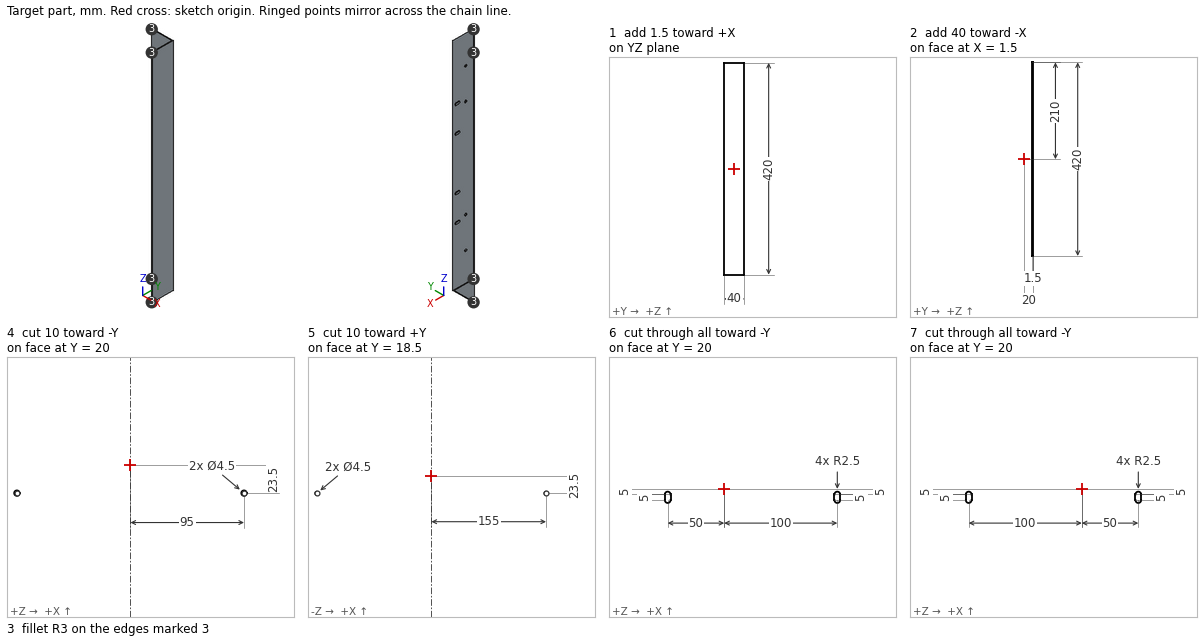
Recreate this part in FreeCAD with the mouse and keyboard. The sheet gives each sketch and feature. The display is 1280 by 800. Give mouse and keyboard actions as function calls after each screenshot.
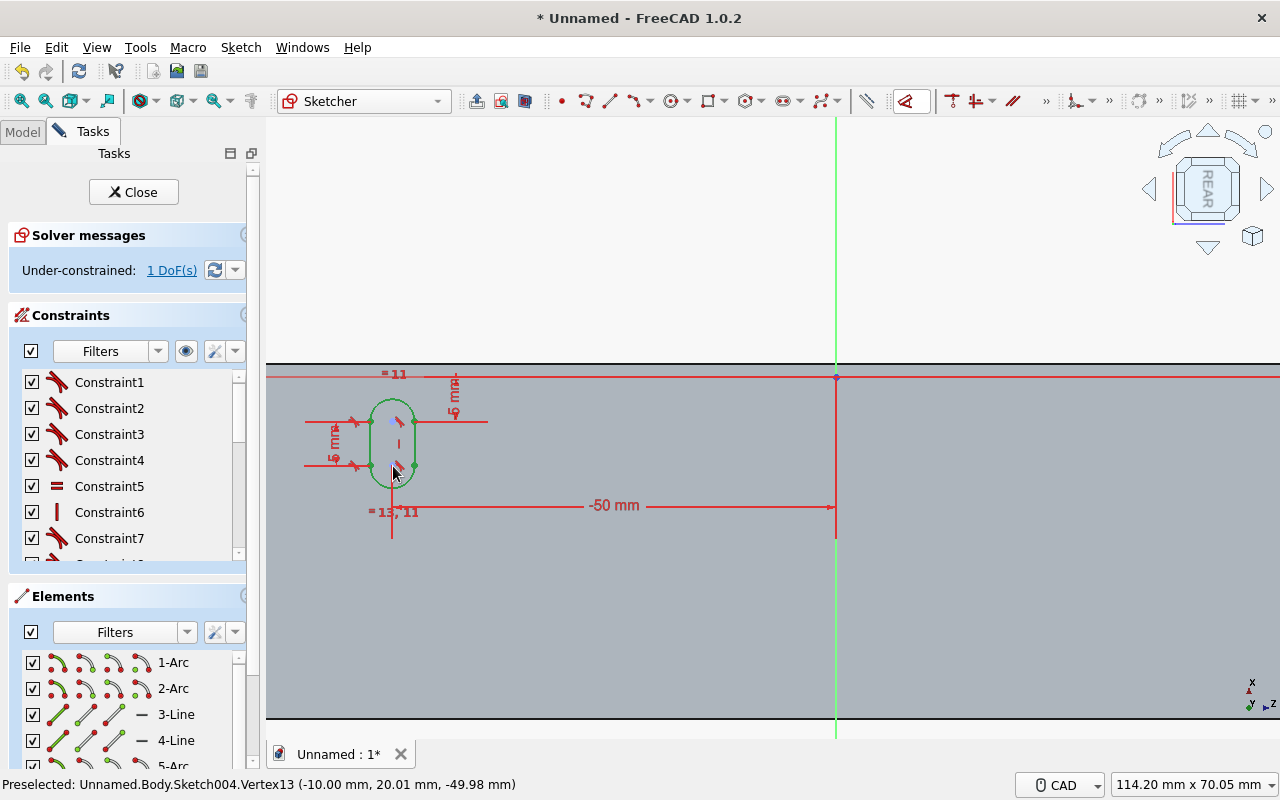
scroll(416, 424, down, 4)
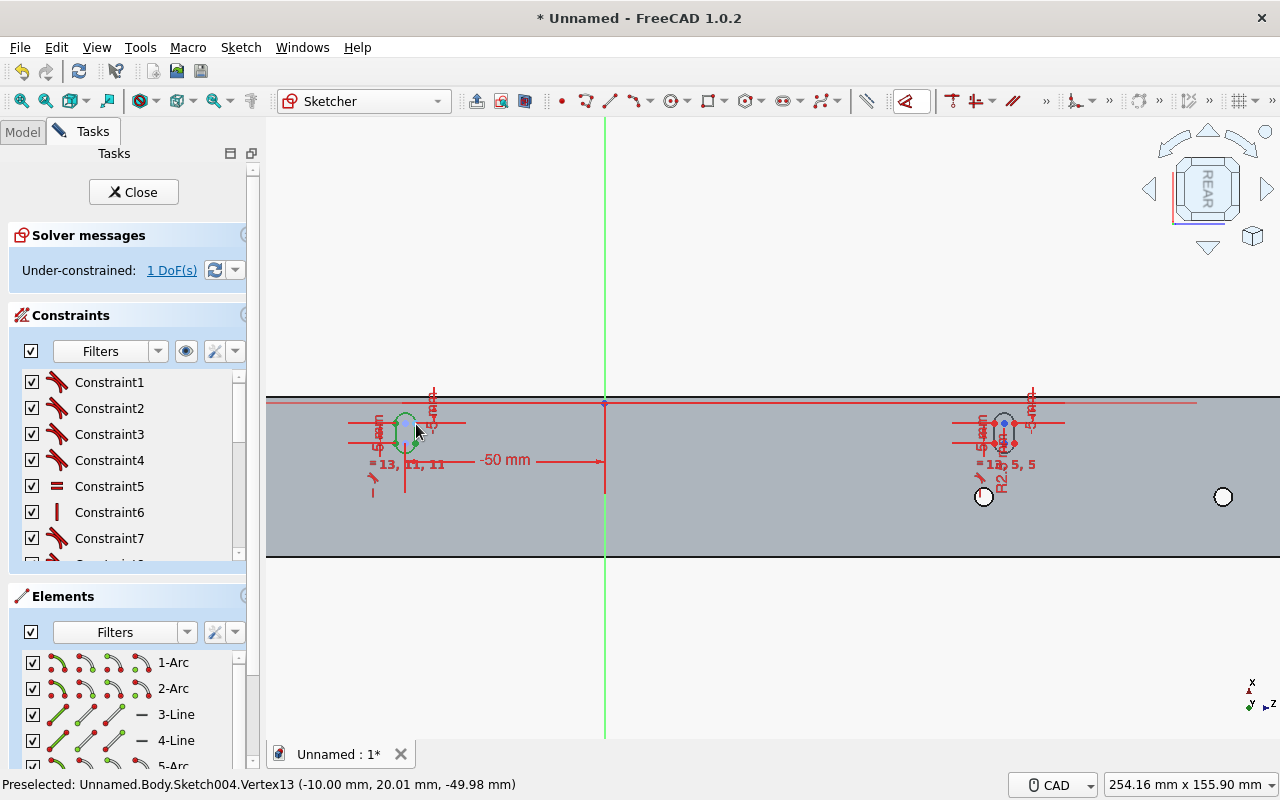
scroll(1004, 443, up, 2)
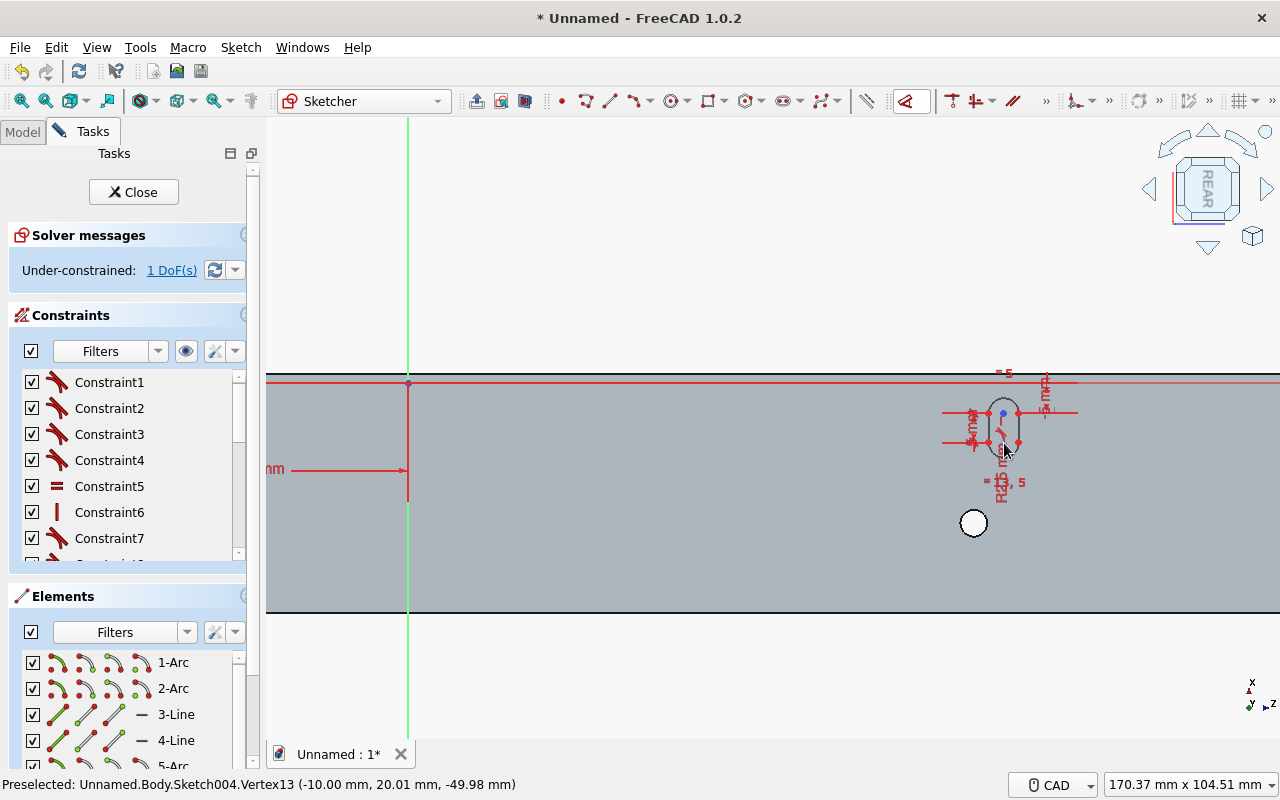
click(1004, 443)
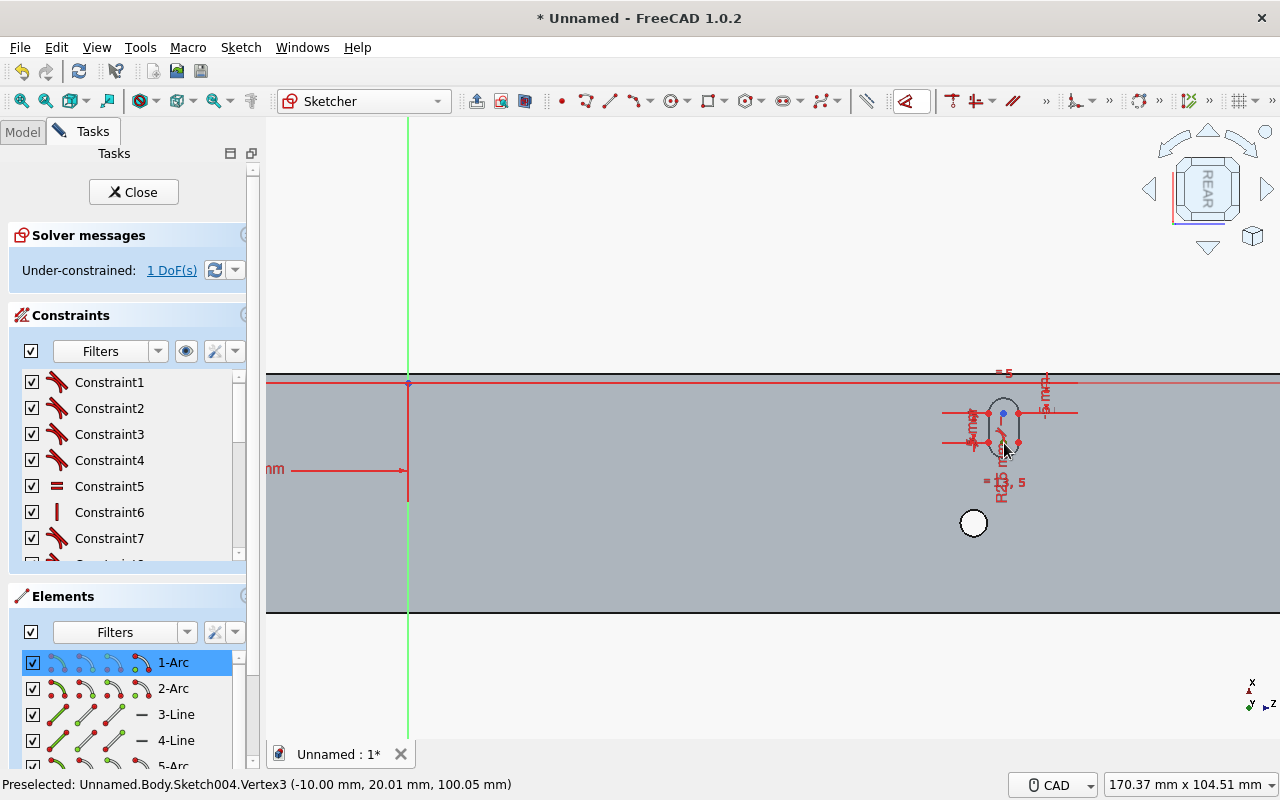
key(l)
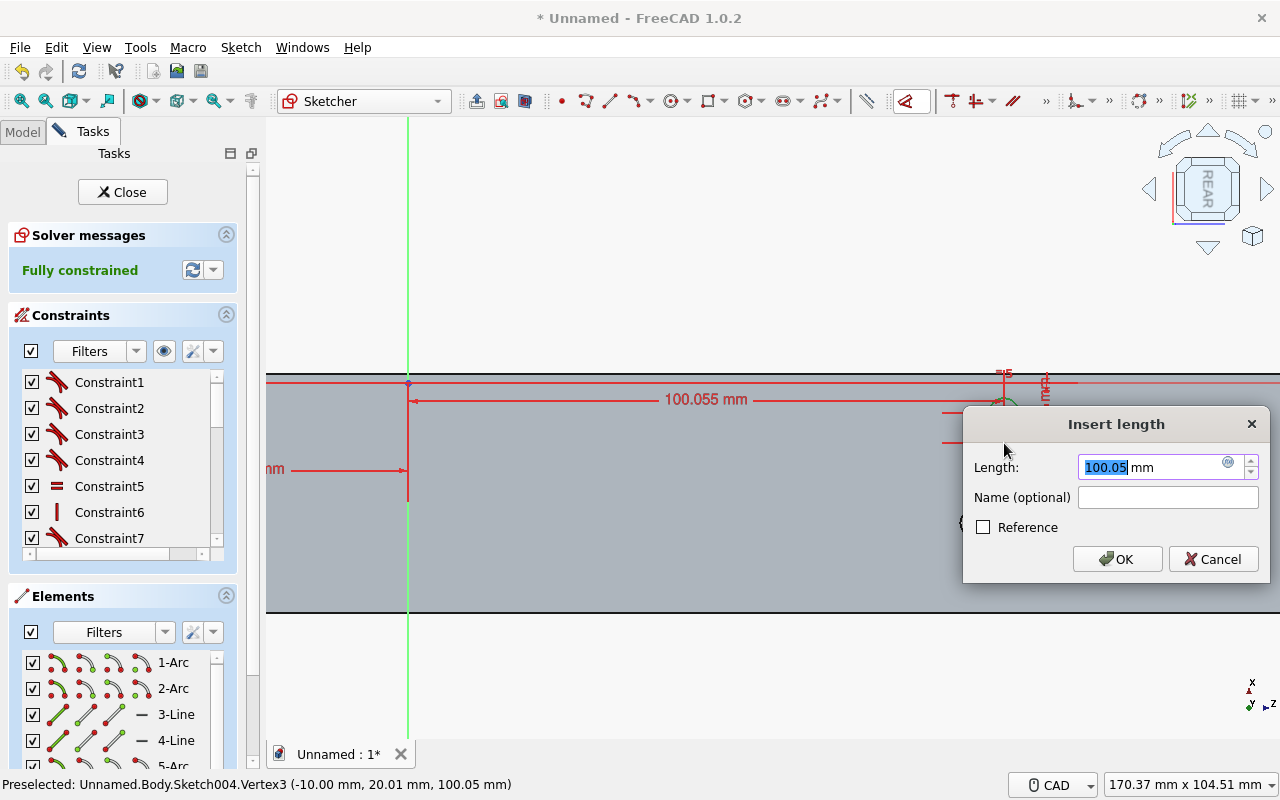
text(100)
key(Return)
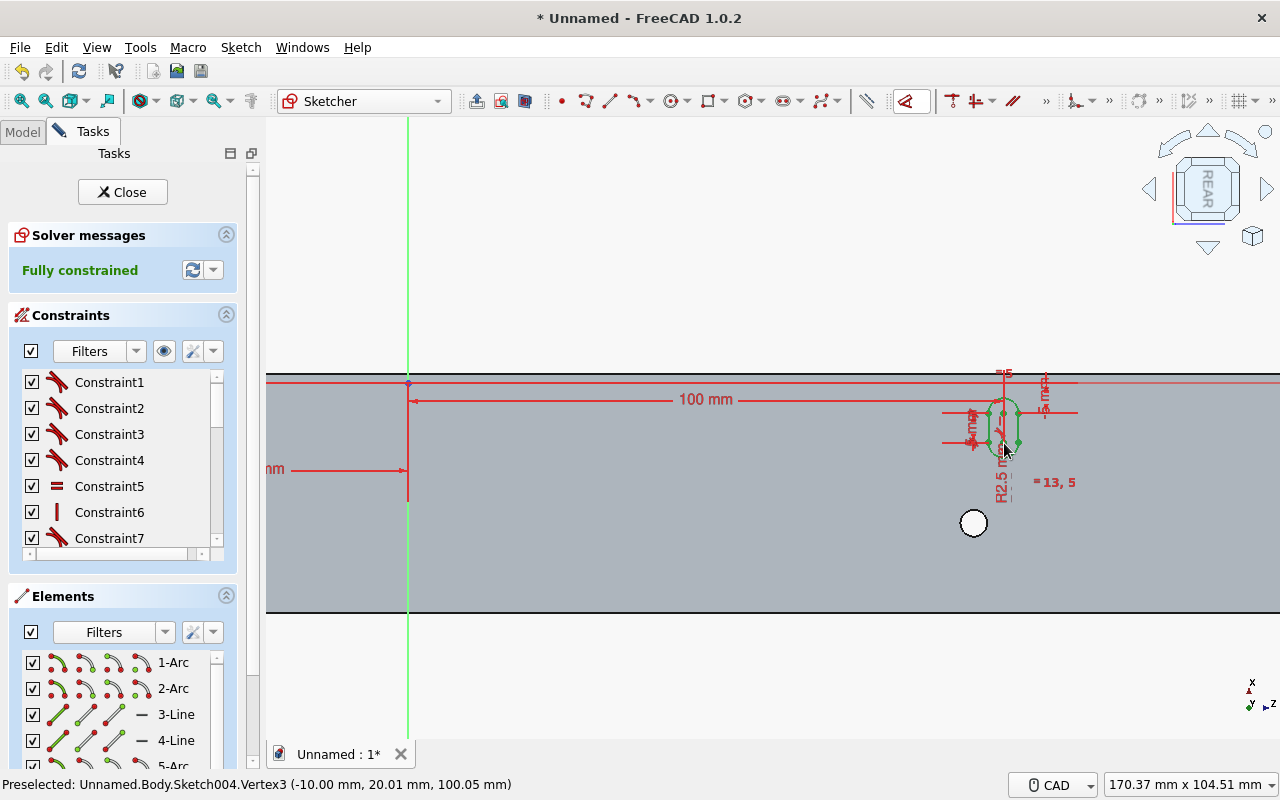
click(123, 192)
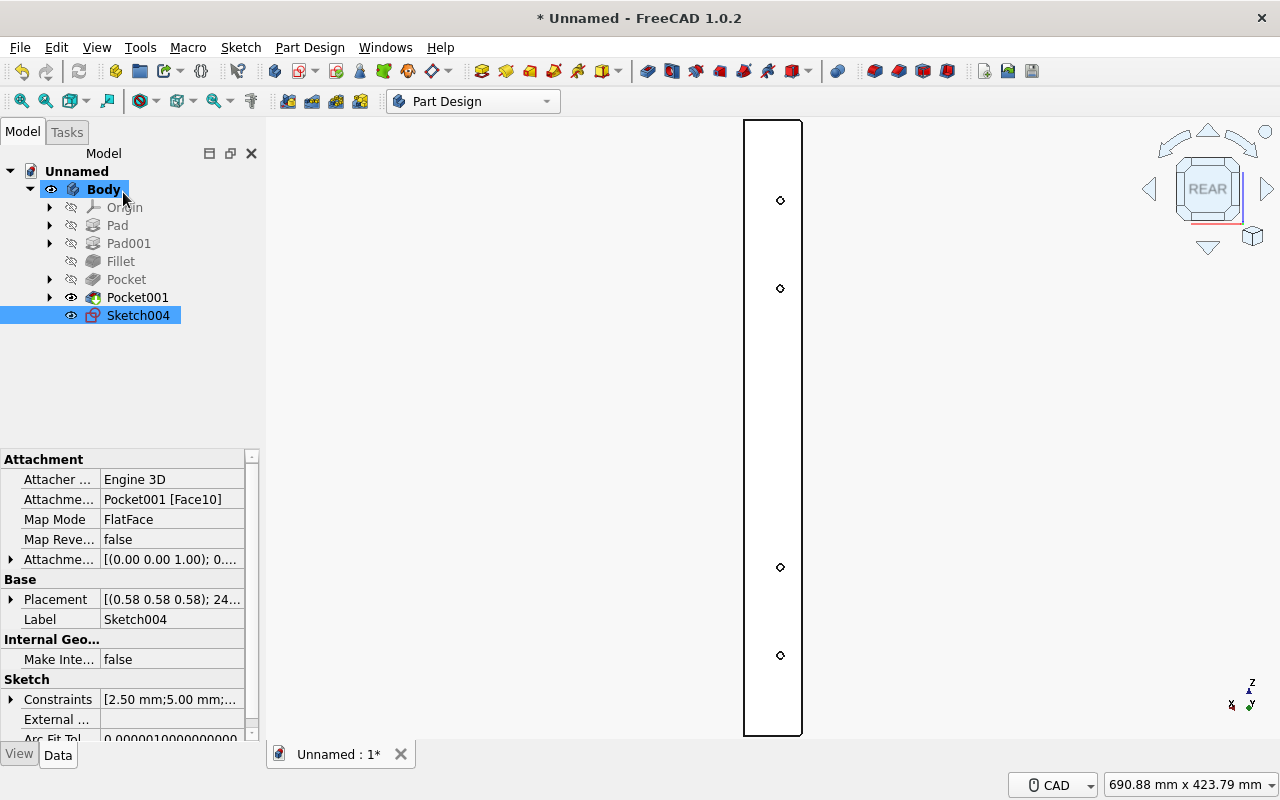
click(648, 72)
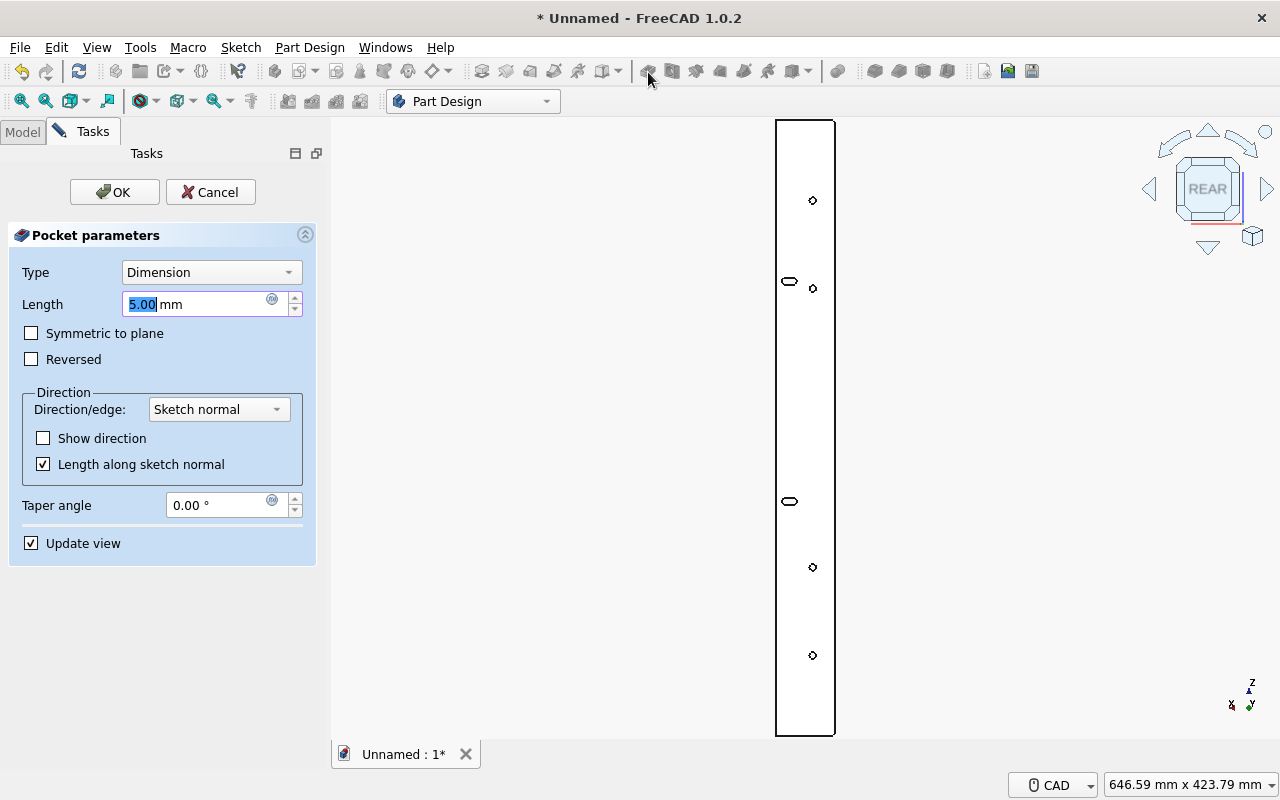
click(212, 272)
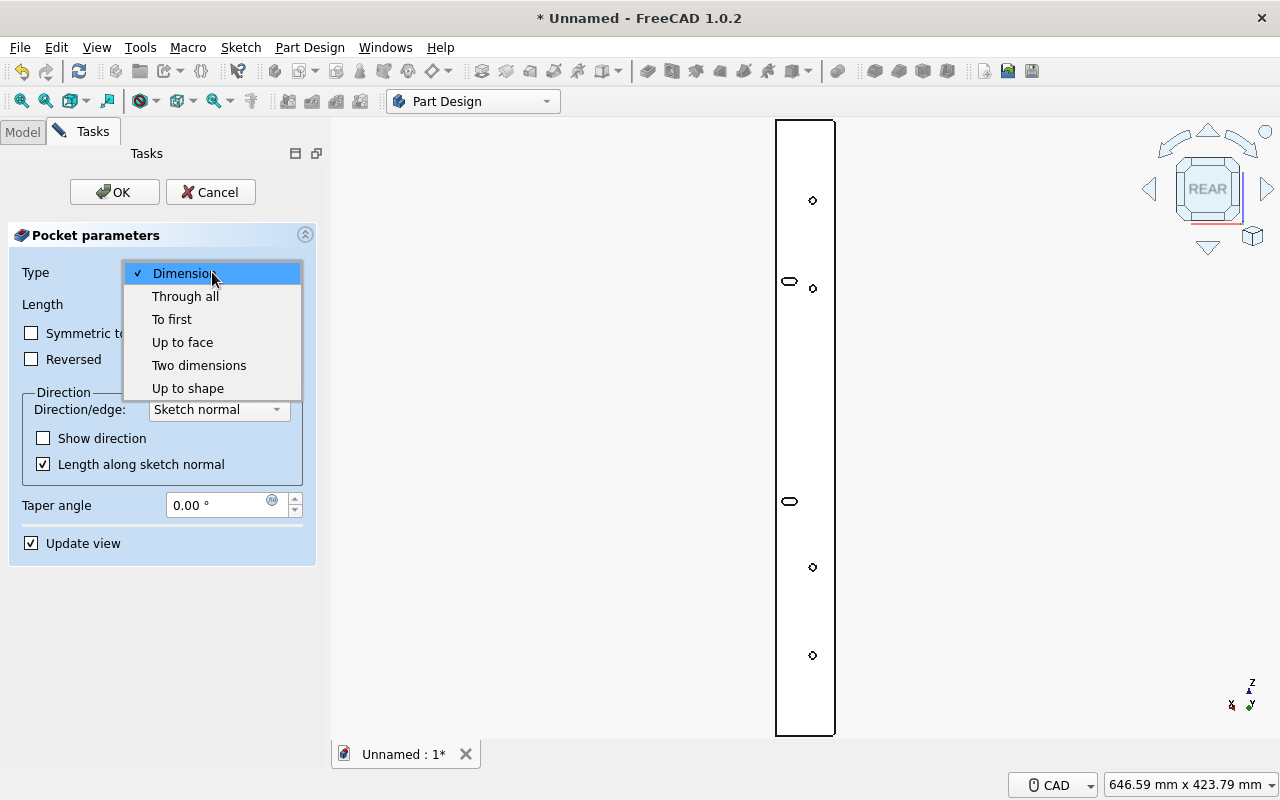
click(212, 296)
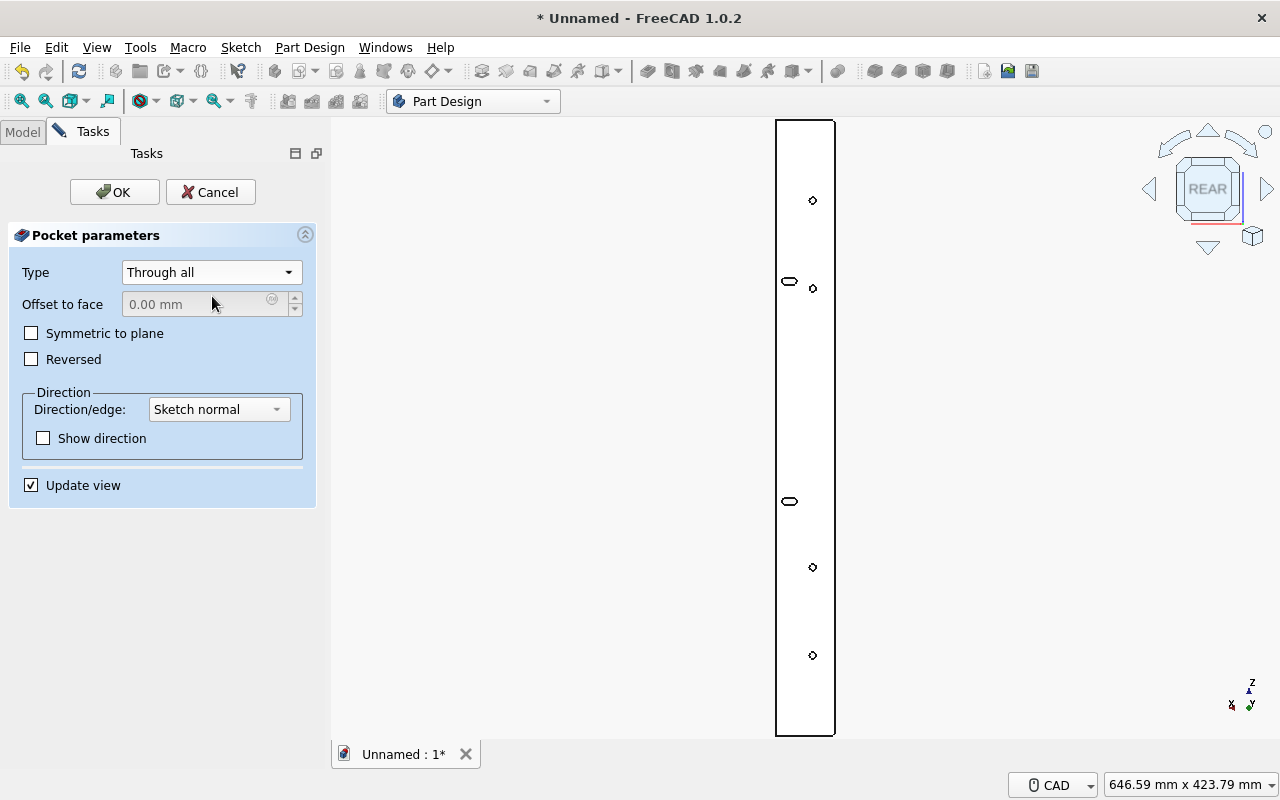
click(115, 192)